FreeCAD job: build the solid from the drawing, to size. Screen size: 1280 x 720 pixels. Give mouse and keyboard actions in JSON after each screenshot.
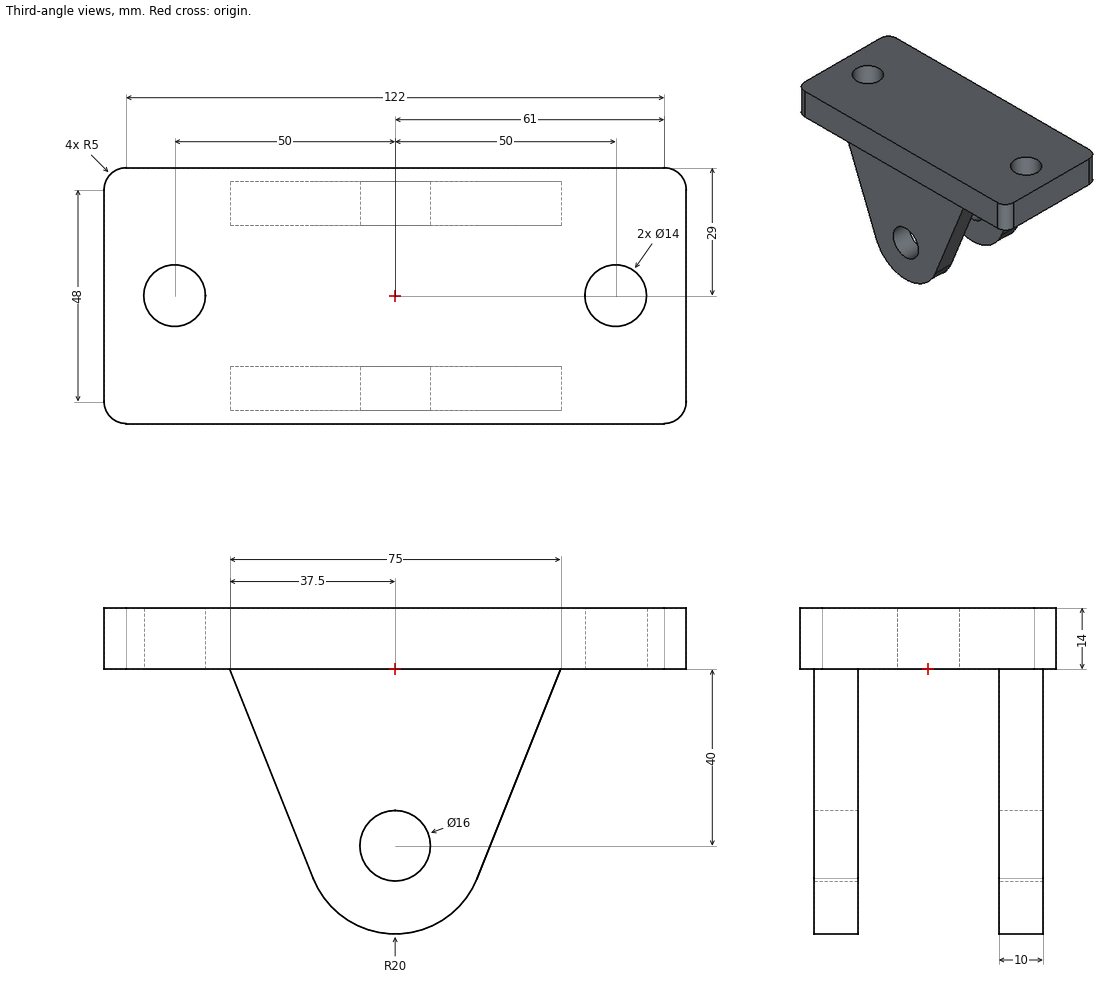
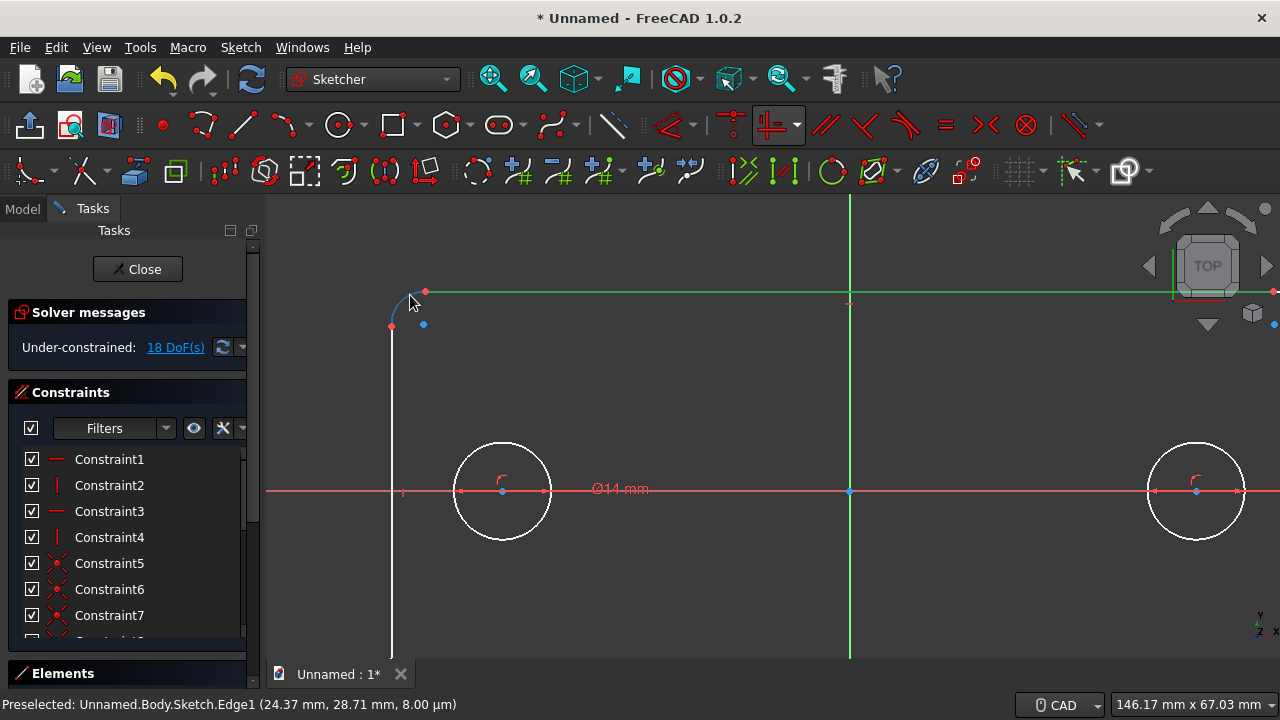
{"action": "left_click", "coordinate": [410, 295]}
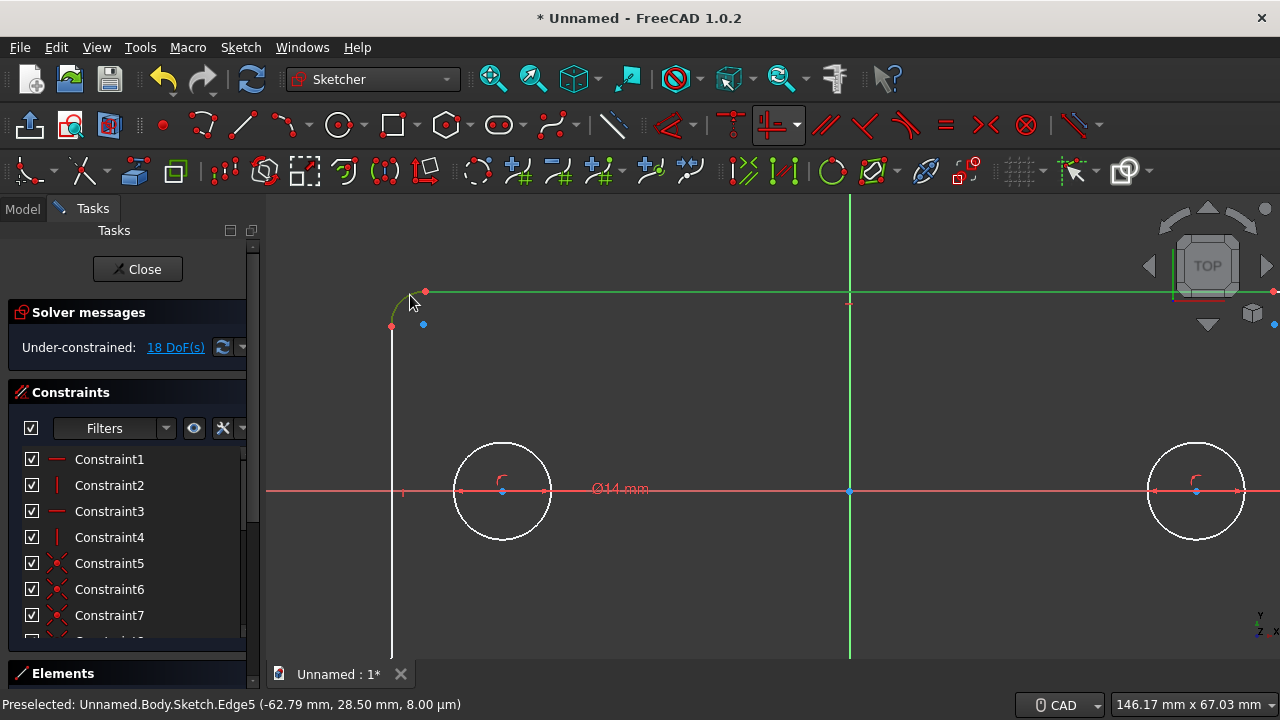
{"action": "left_click", "coordinate": [906, 126]}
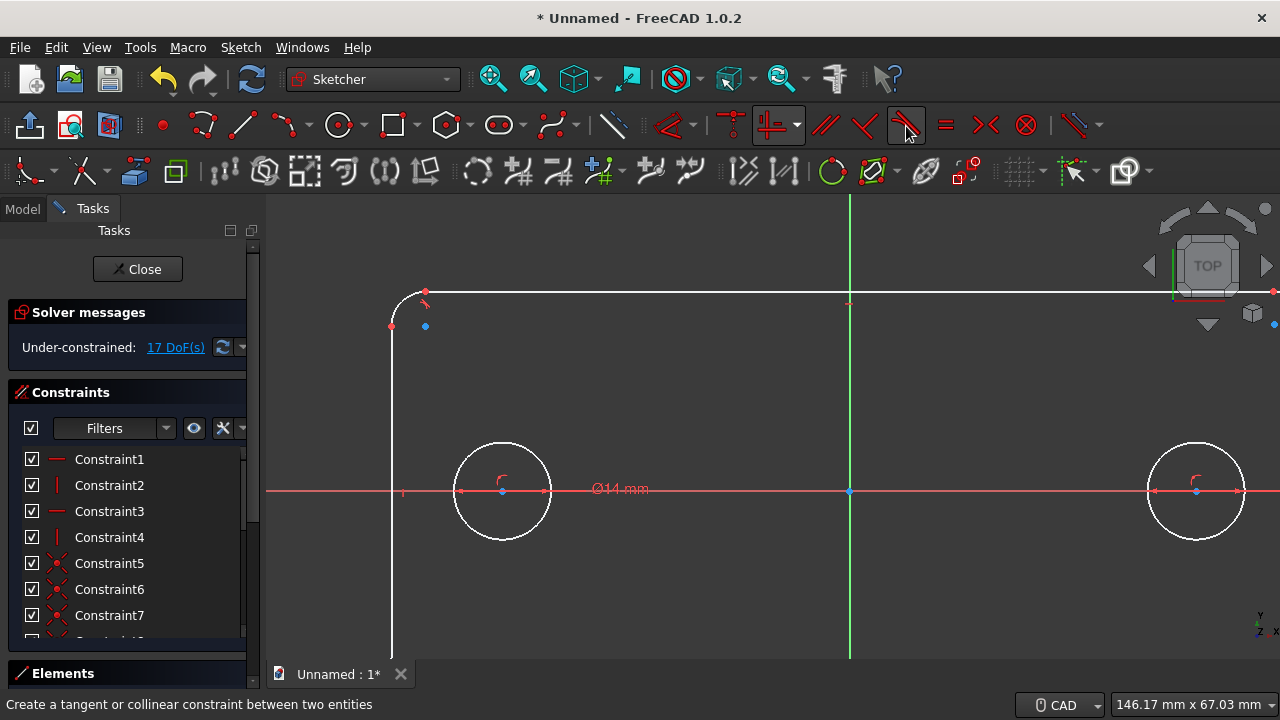
{"action": "left_click", "coordinate": [1019, 292]}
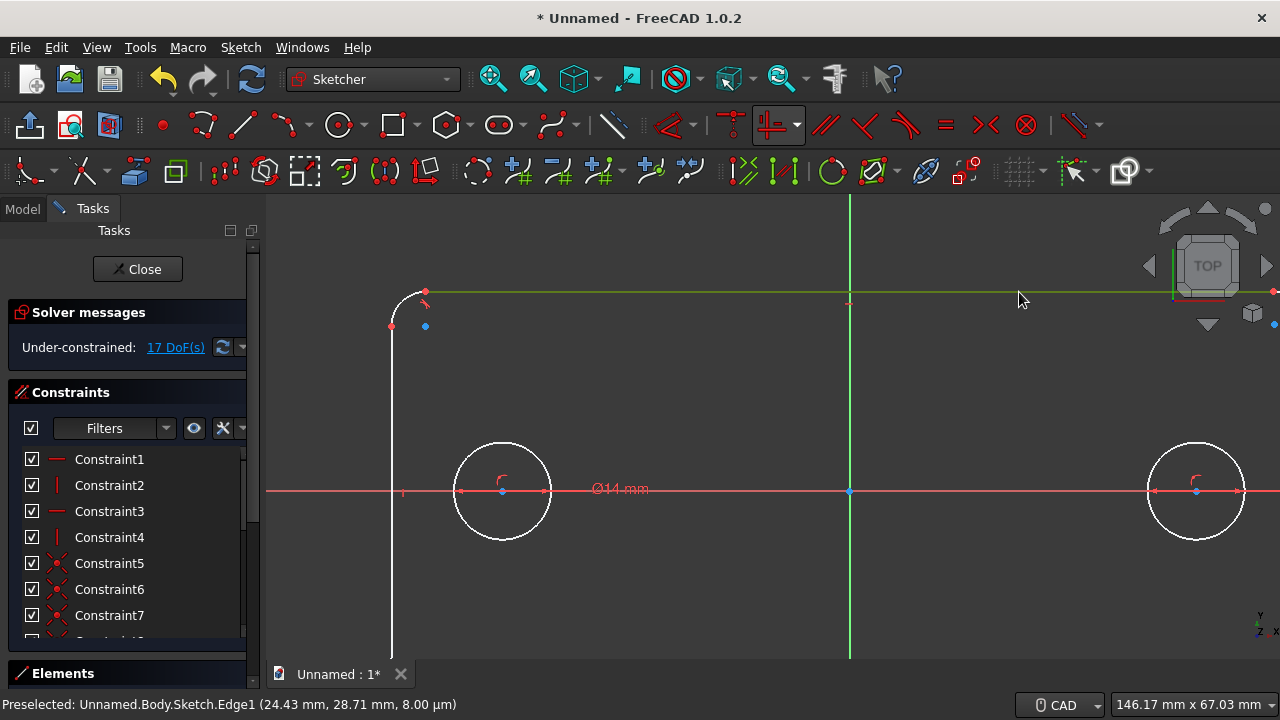
{"action": "scroll", "coordinate": [410, 295], "scroll_direction": "down", "scroll_amount": 2}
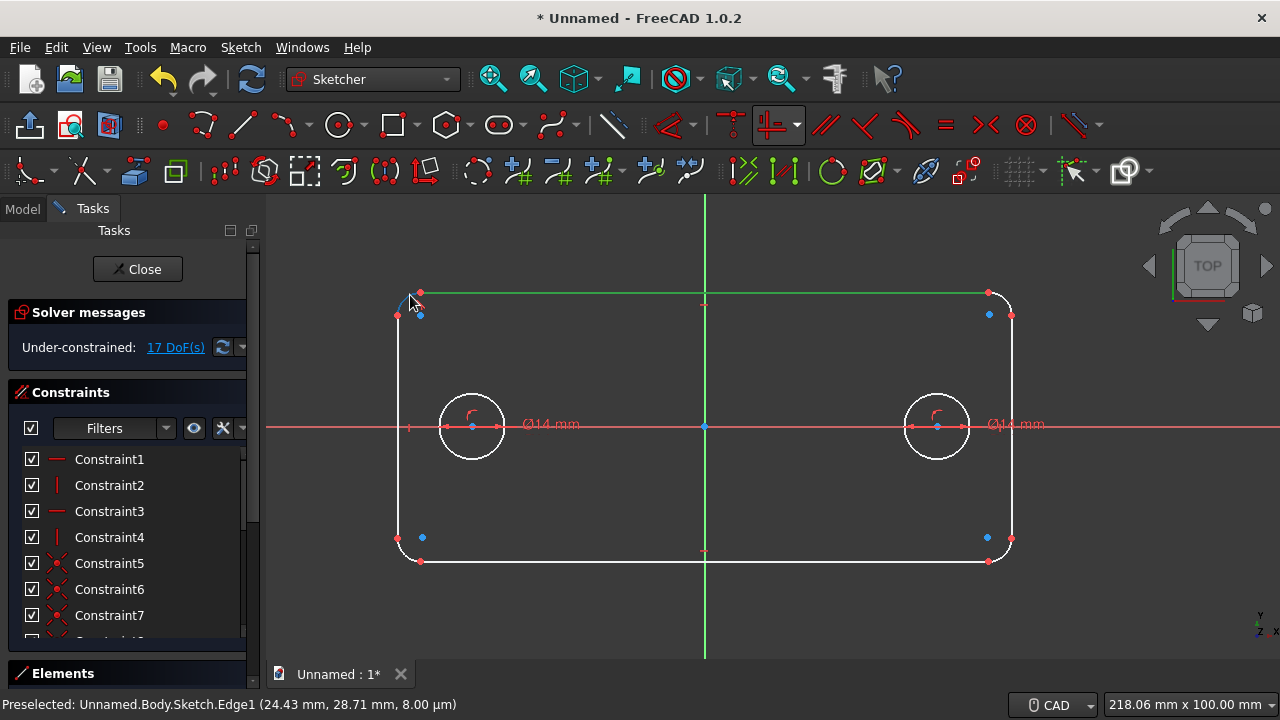
{"action": "scroll", "coordinate": [1009, 305], "scroll_direction": "up", "scroll_amount": 2}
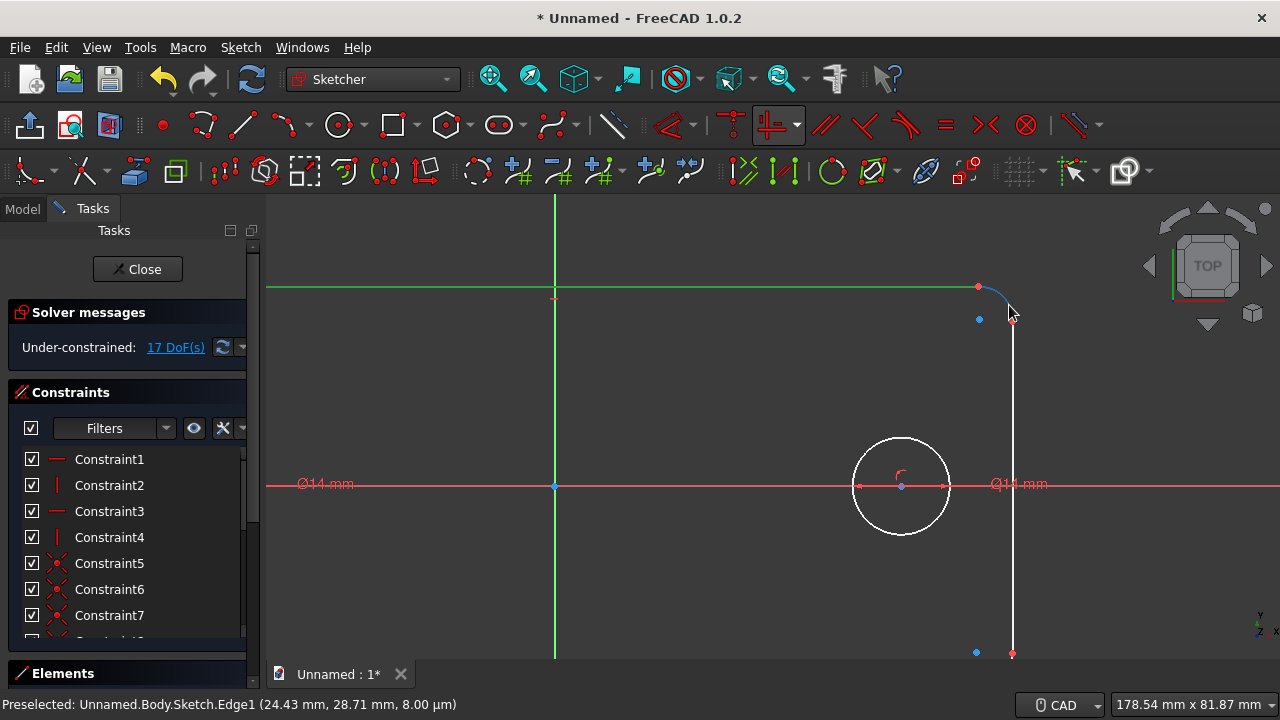
{"action": "left_click", "coordinate": [1009, 305]}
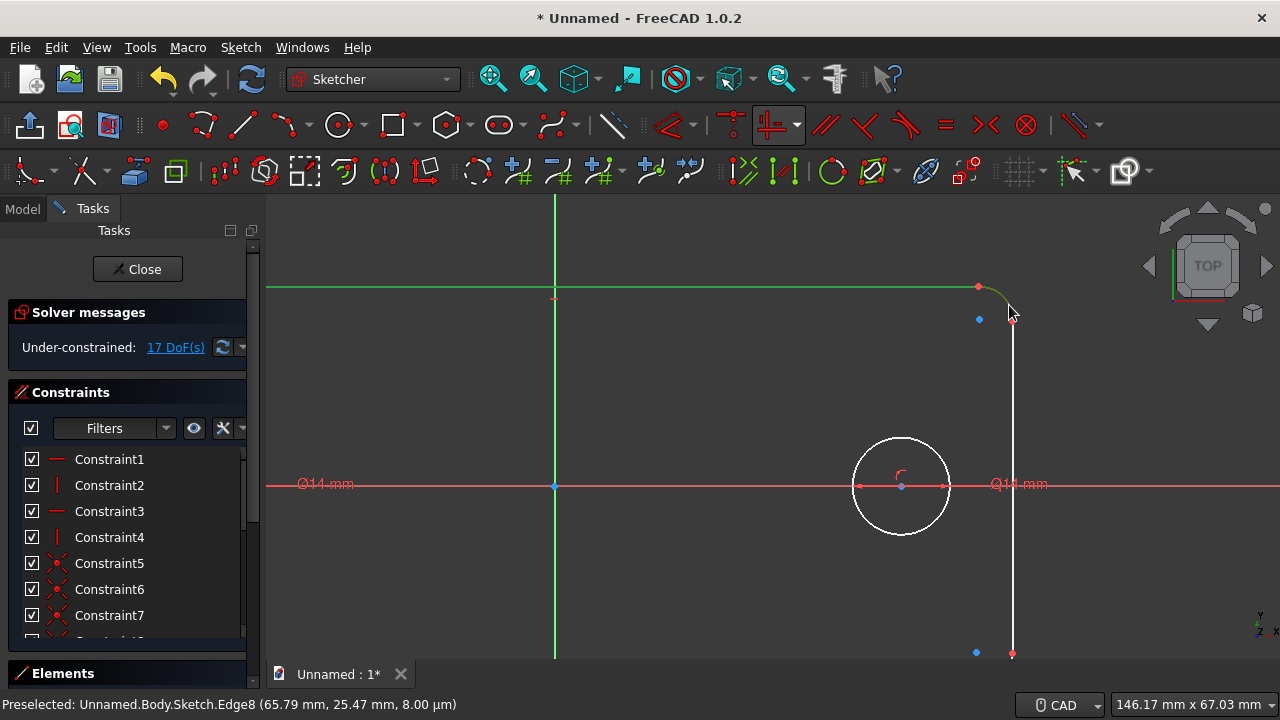
{"action": "left_click", "coordinate": [906, 126]}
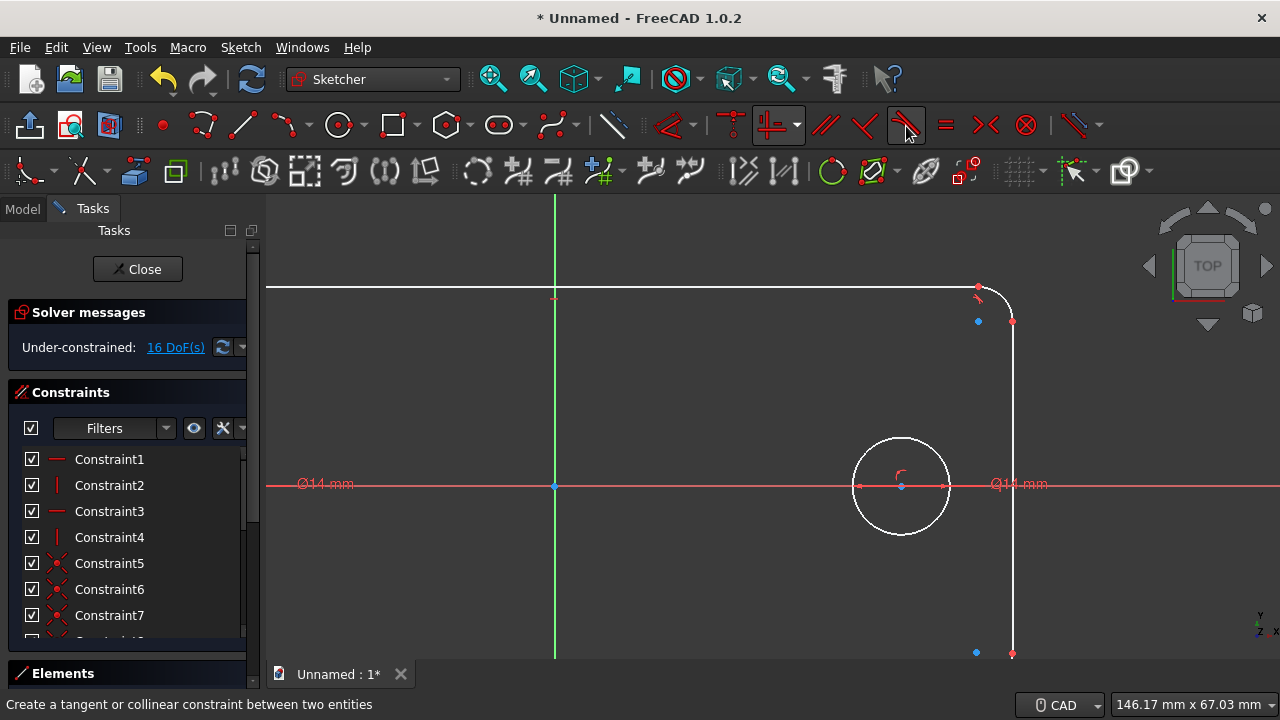
{"action": "scroll", "coordinate": [1009, 305], "scroll_direction": "down", "scroll_amount": 2}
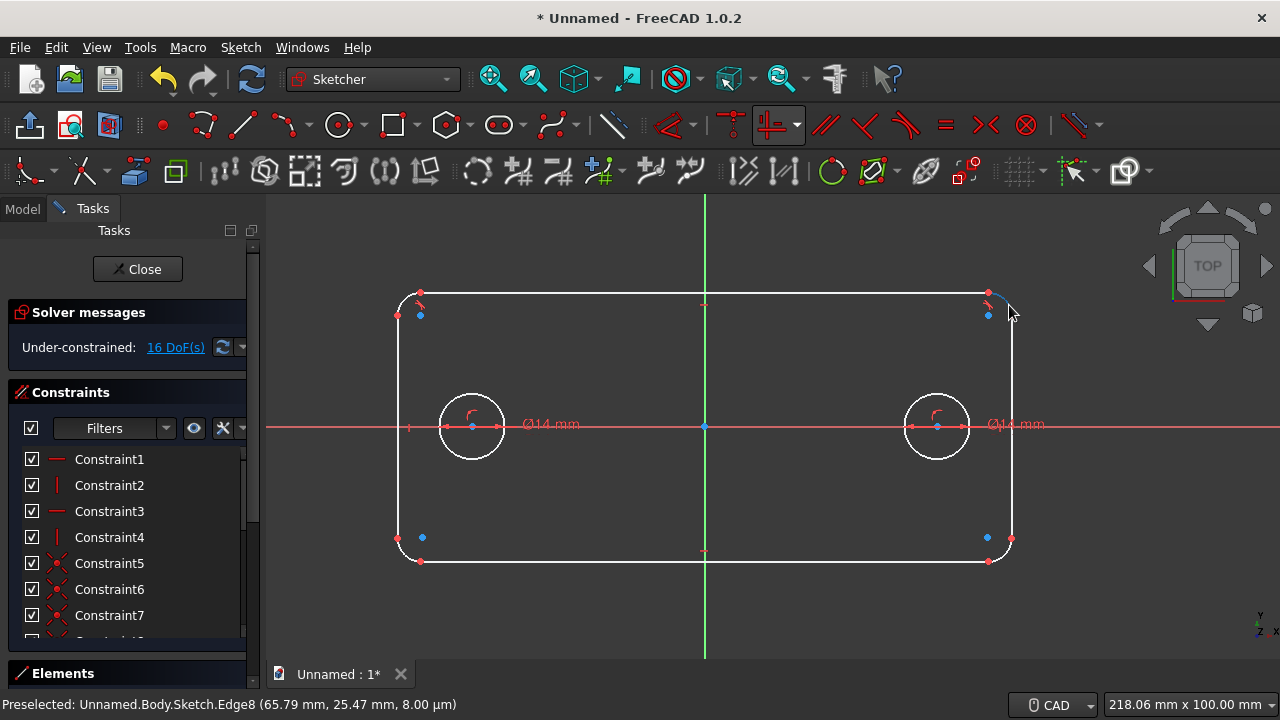
{"action": "left_click", "coordinate": [398, 383]}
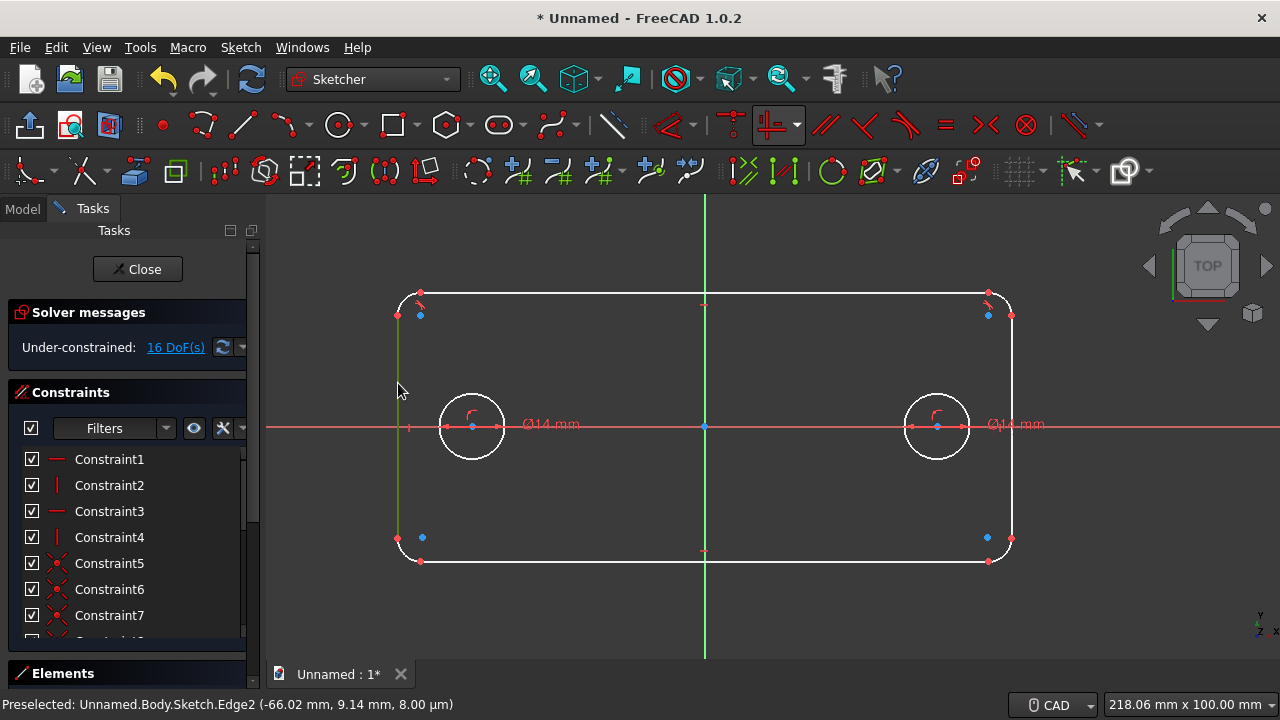
{"action": "scroll", "coordinate": [410, 296], "scroll_direction": "up", "scroll_amount": 2}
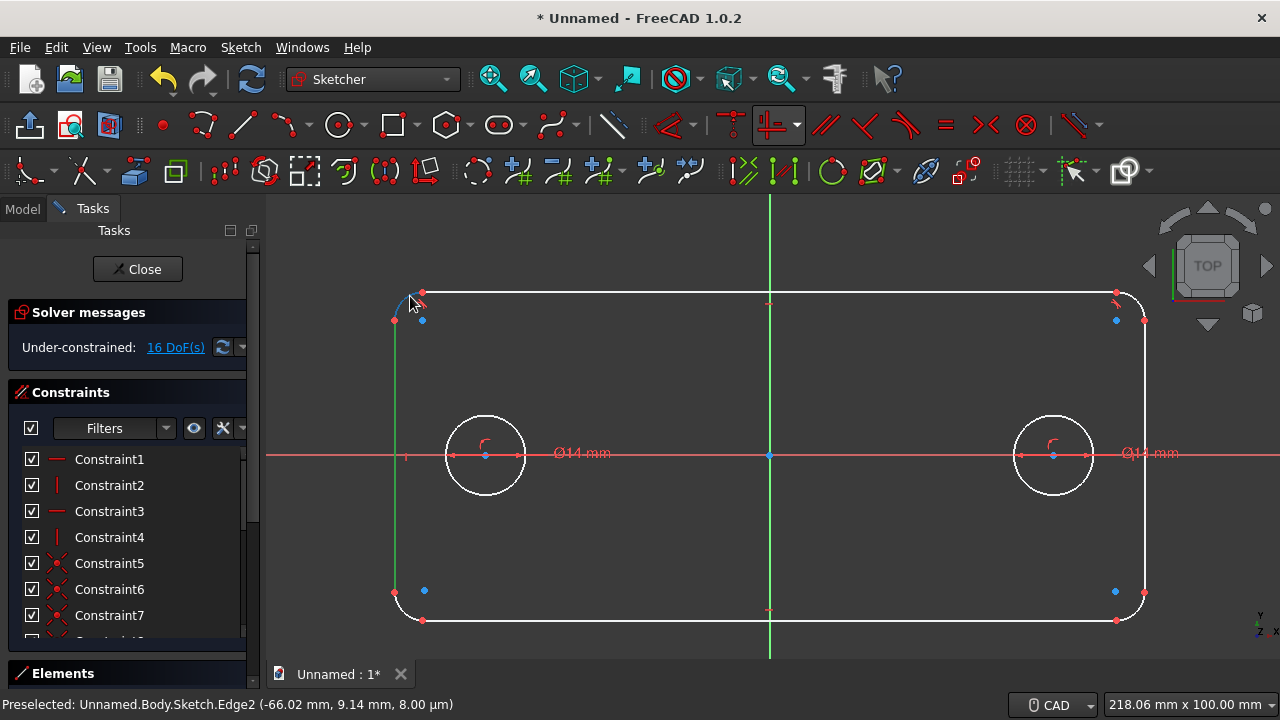
{"action": "left_click", "coordinate": [410, 295]}